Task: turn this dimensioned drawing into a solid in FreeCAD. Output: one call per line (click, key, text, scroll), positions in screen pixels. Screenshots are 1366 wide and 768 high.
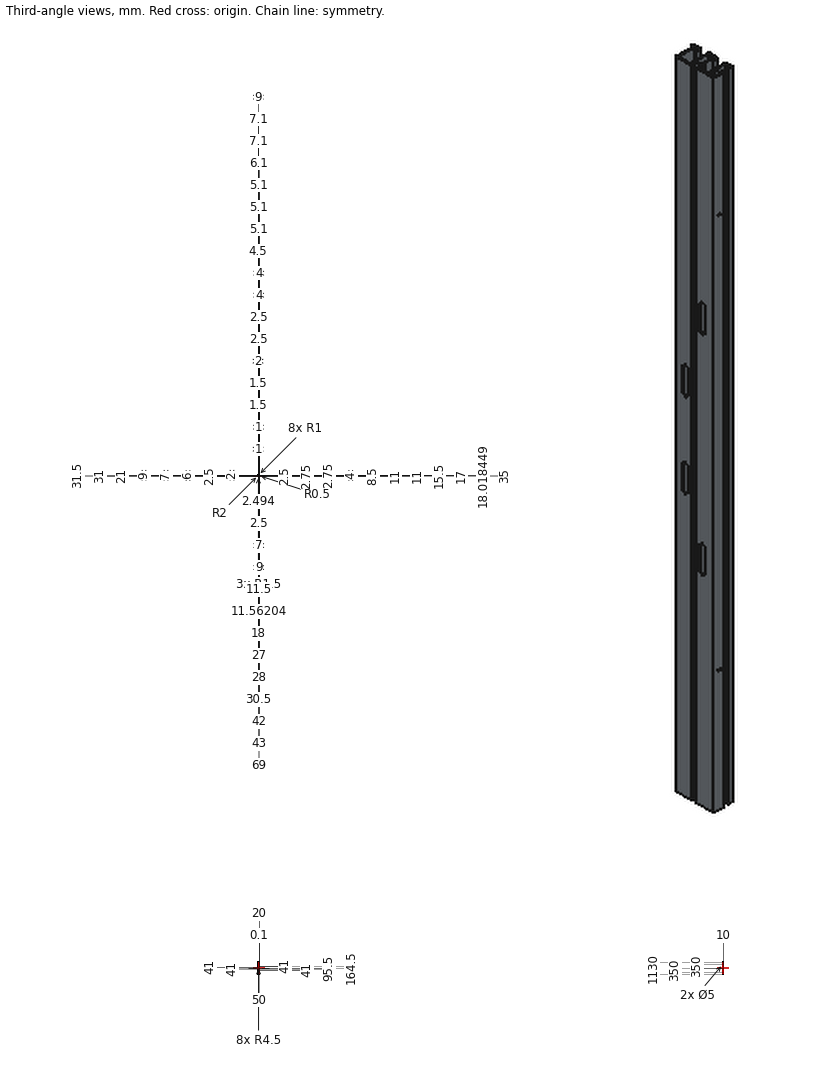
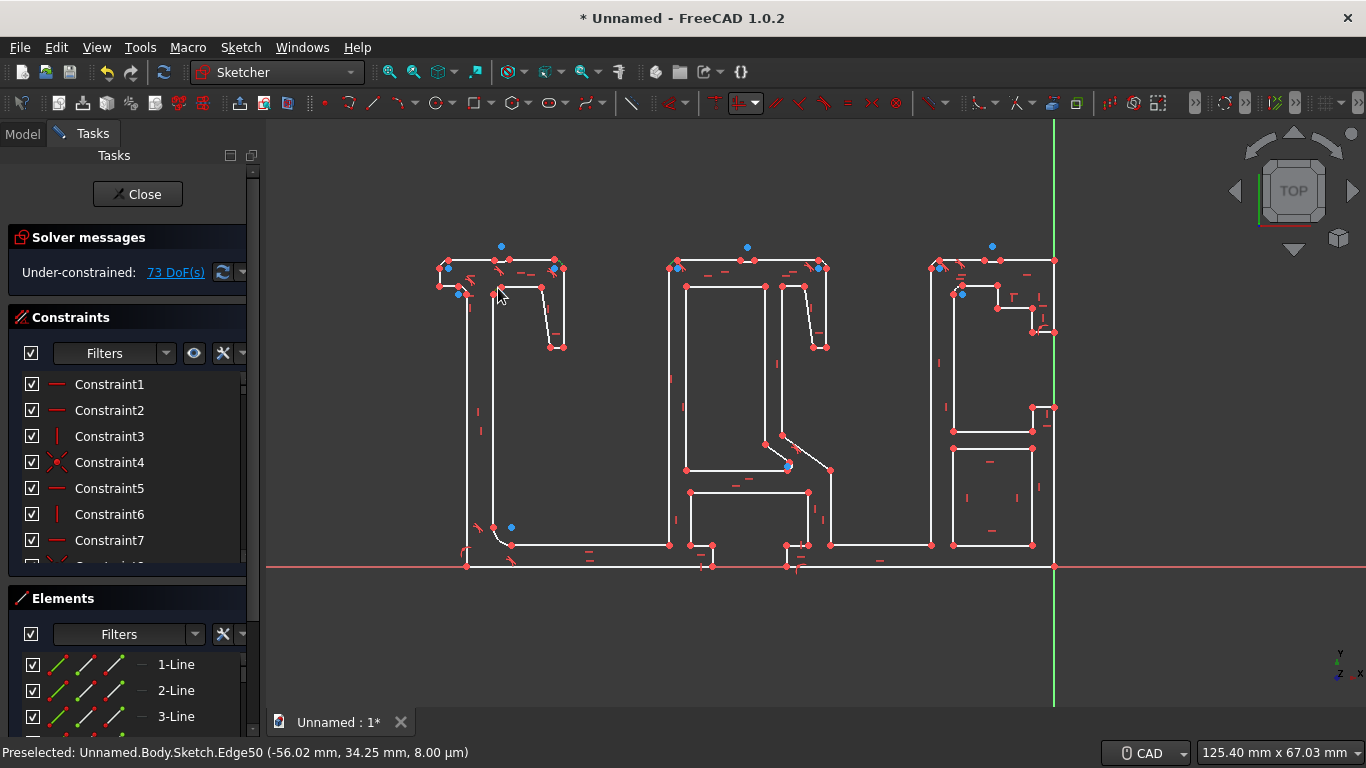
scroll(444, 261, up, 7)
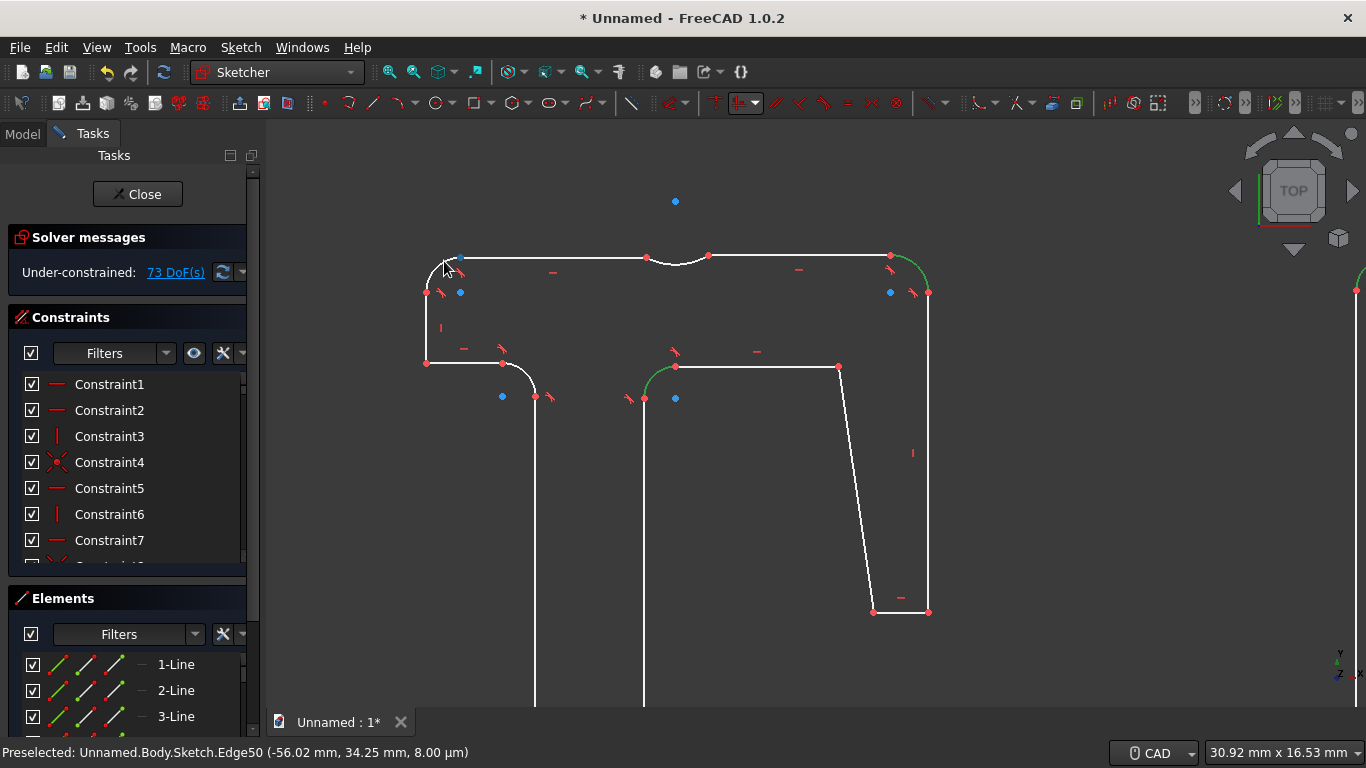
click(445, 261)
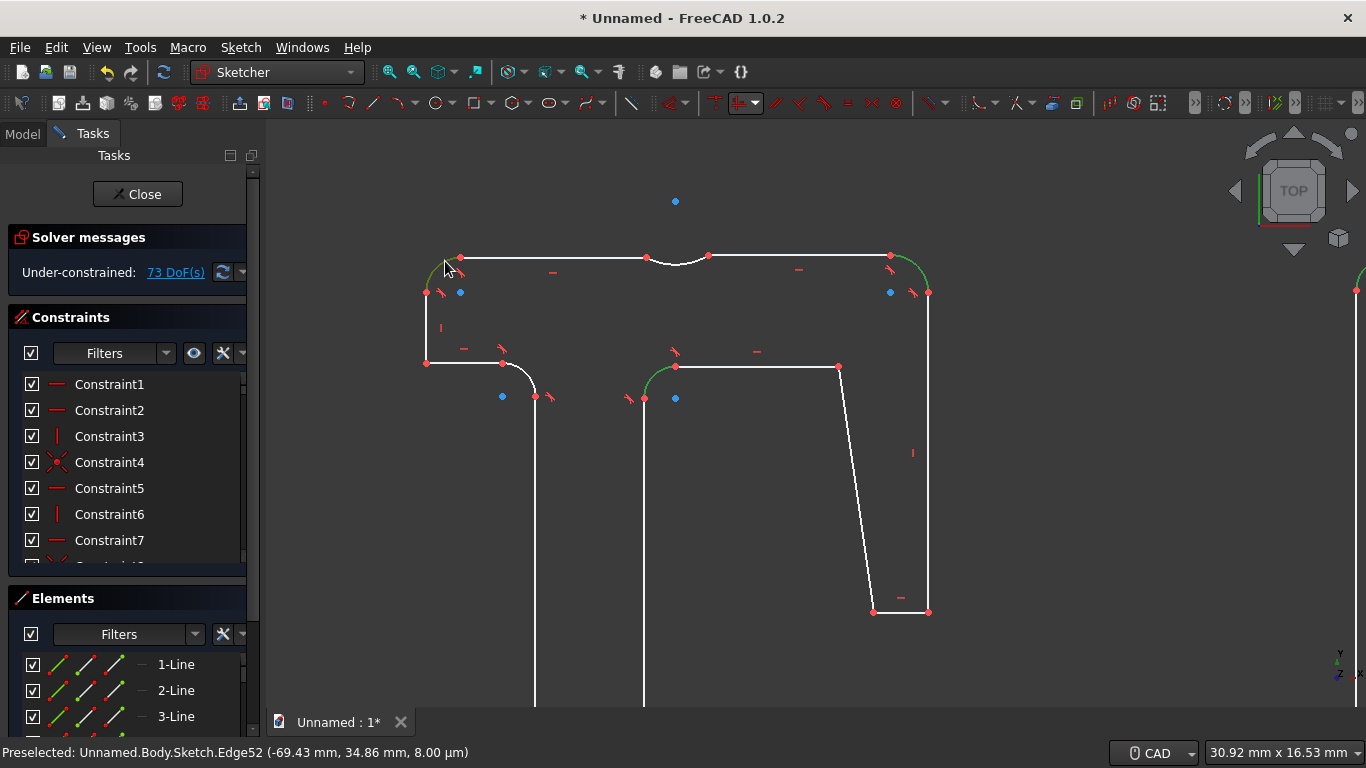
click(532, 381)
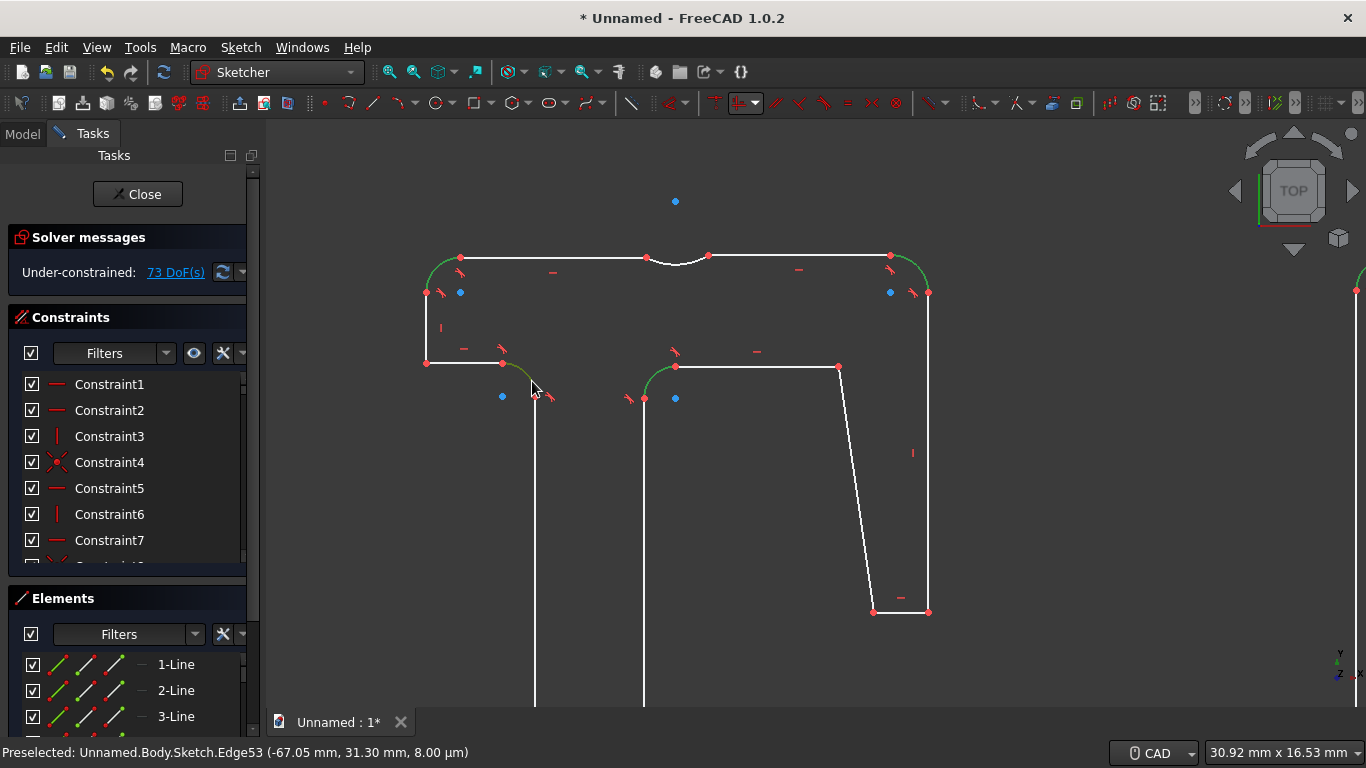
scroll(444, 261, down, 7)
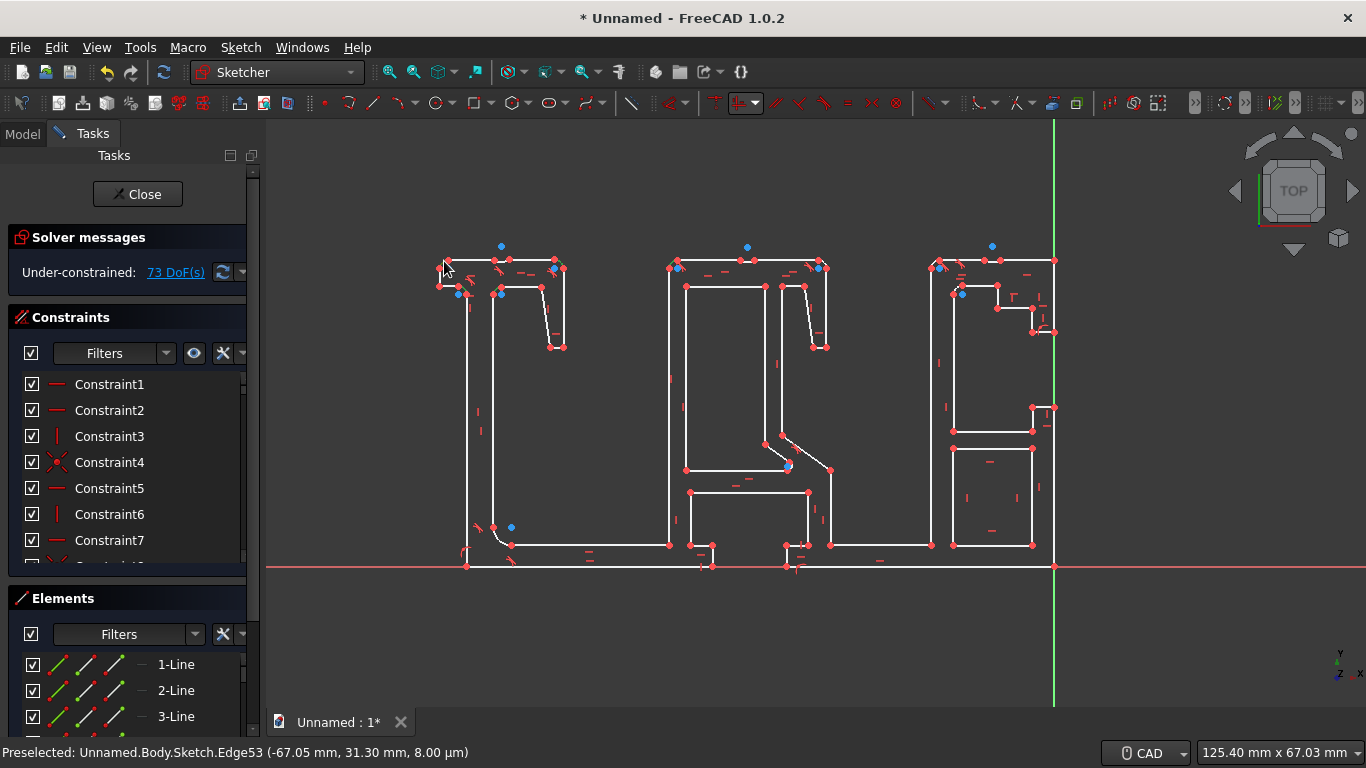
scroll(958, 287, up, 7)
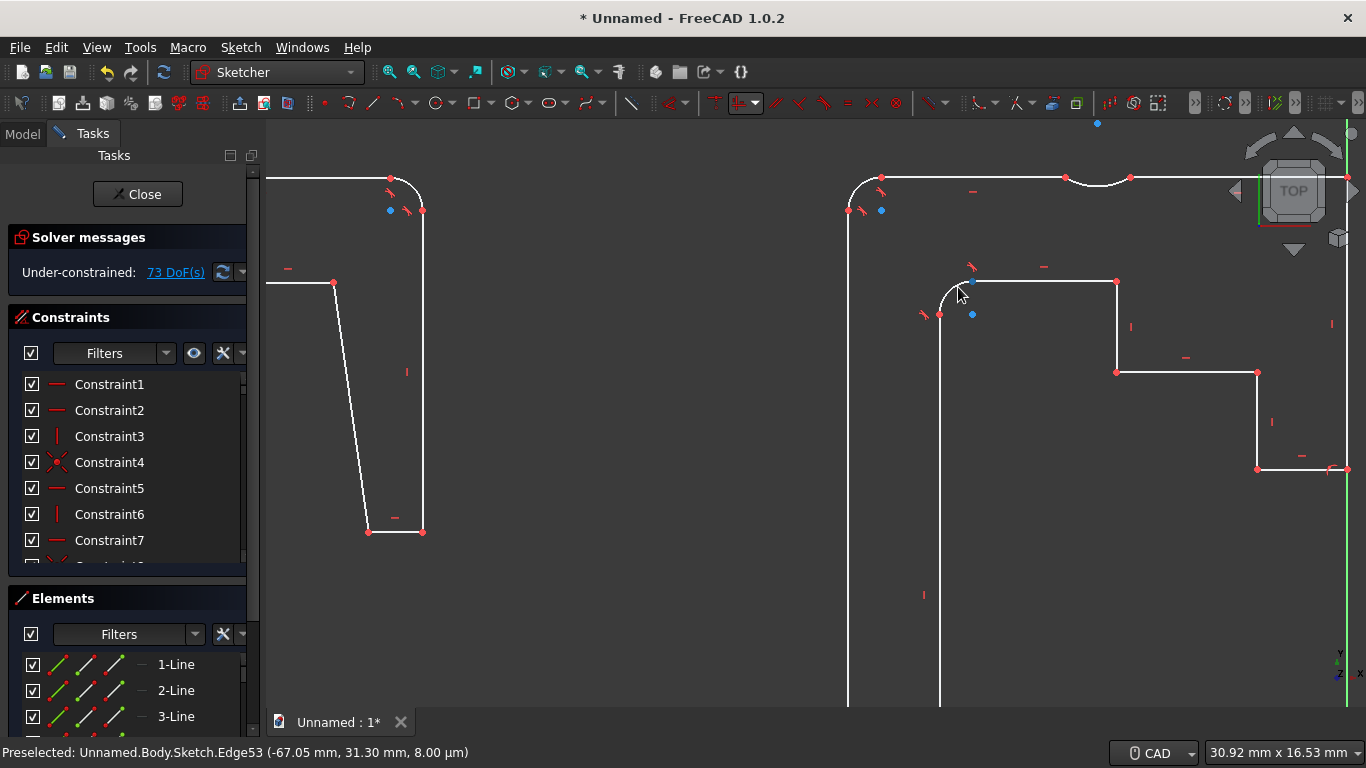
click(958, 285)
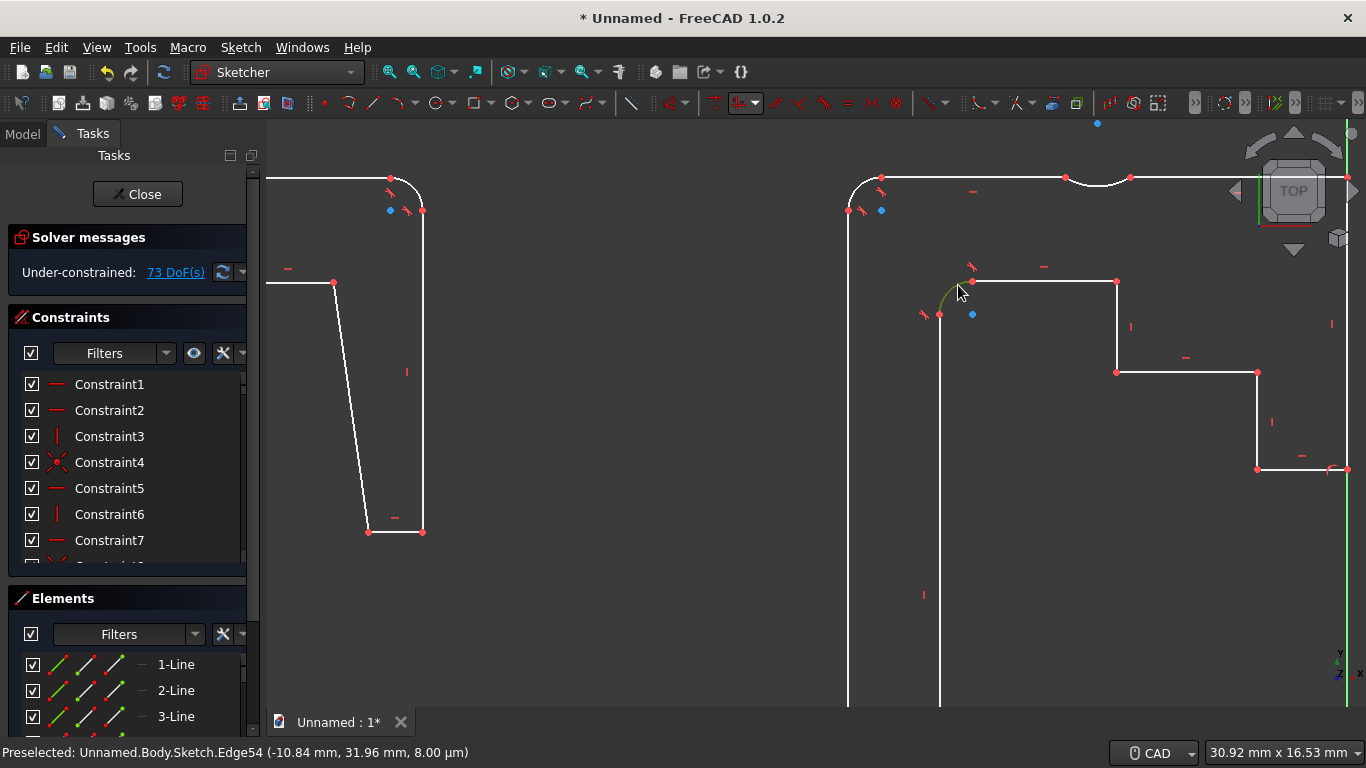
click(867, 181)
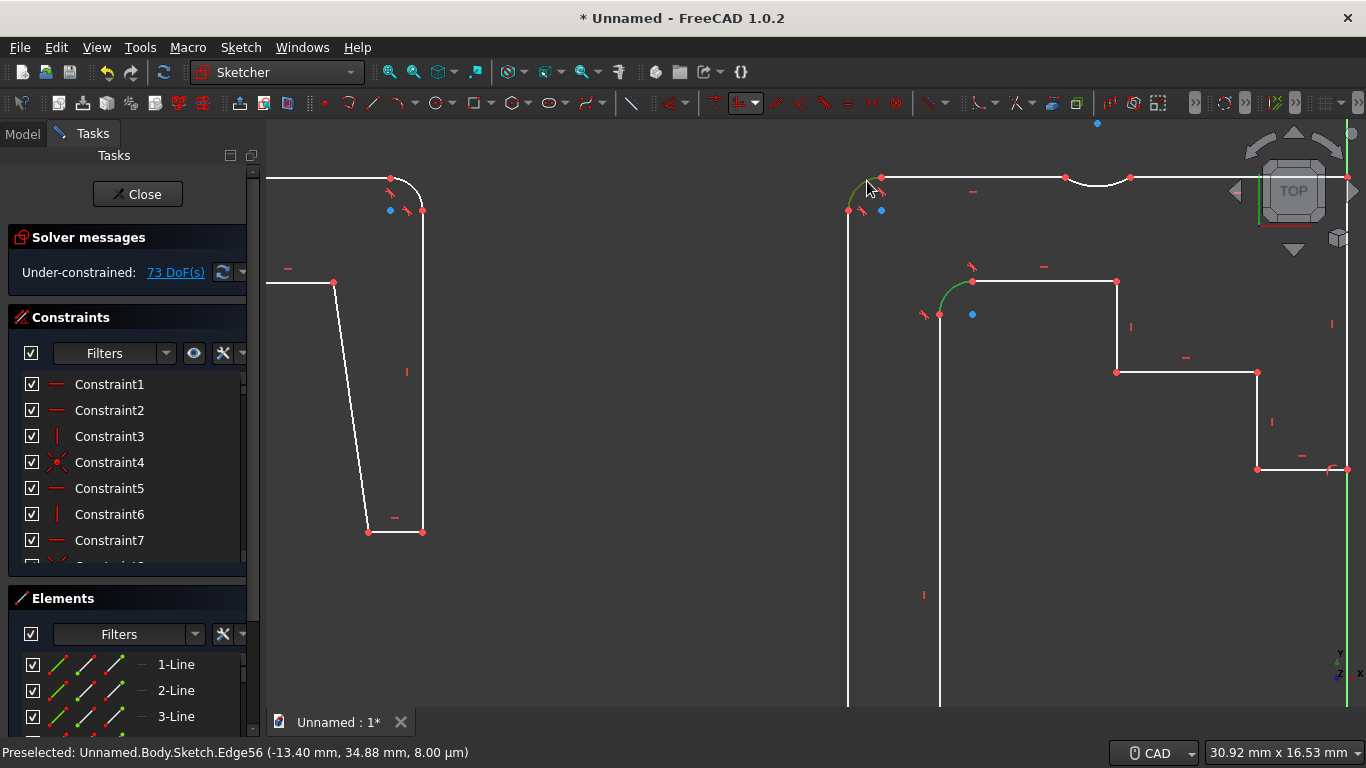
click(419, 196)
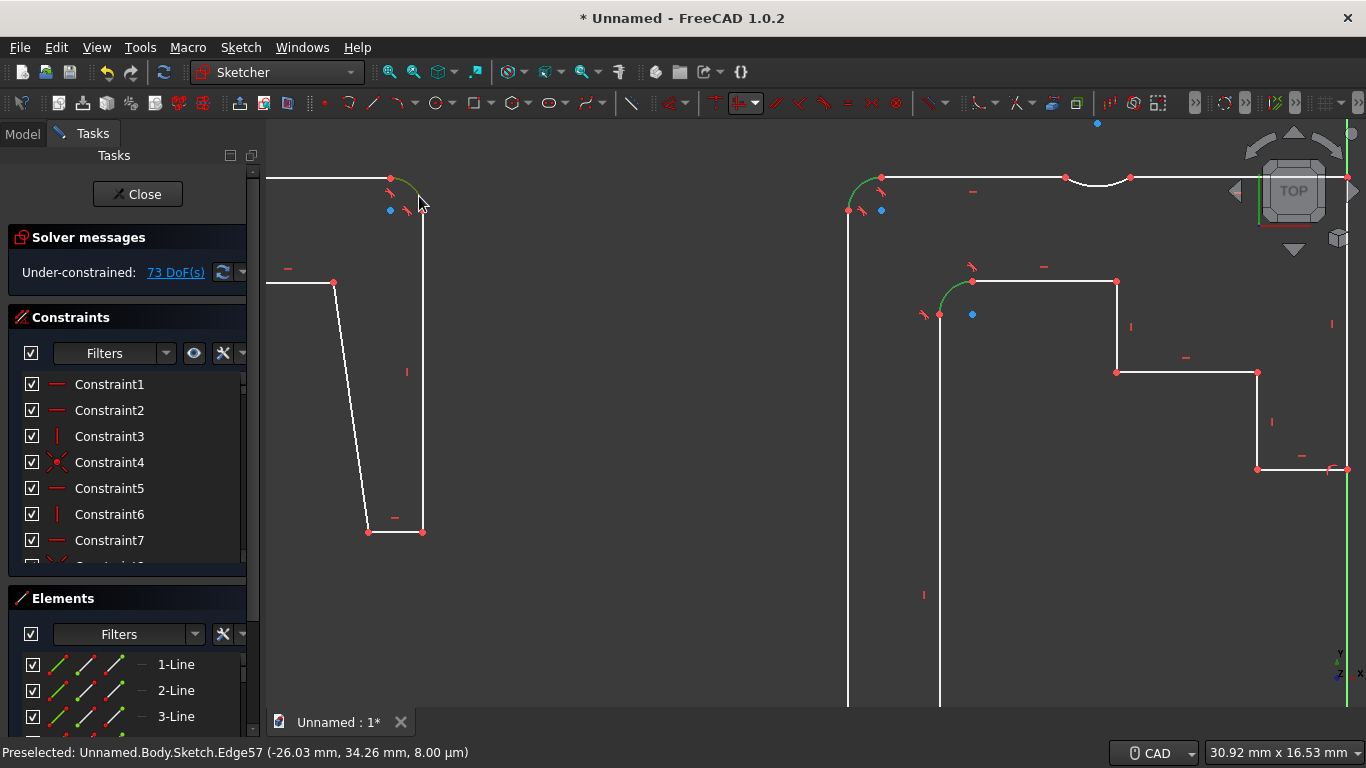
click(848, 104)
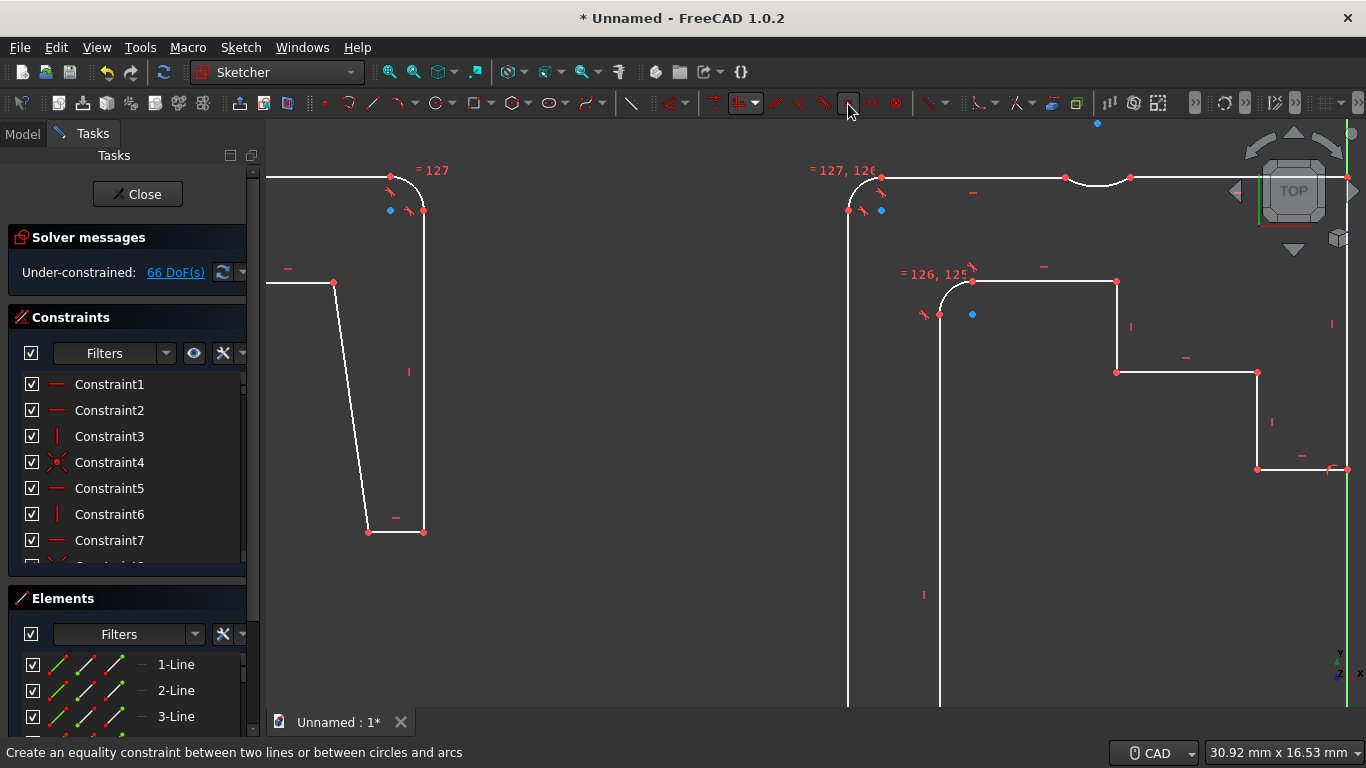
scroll(959, 287, down, 7)